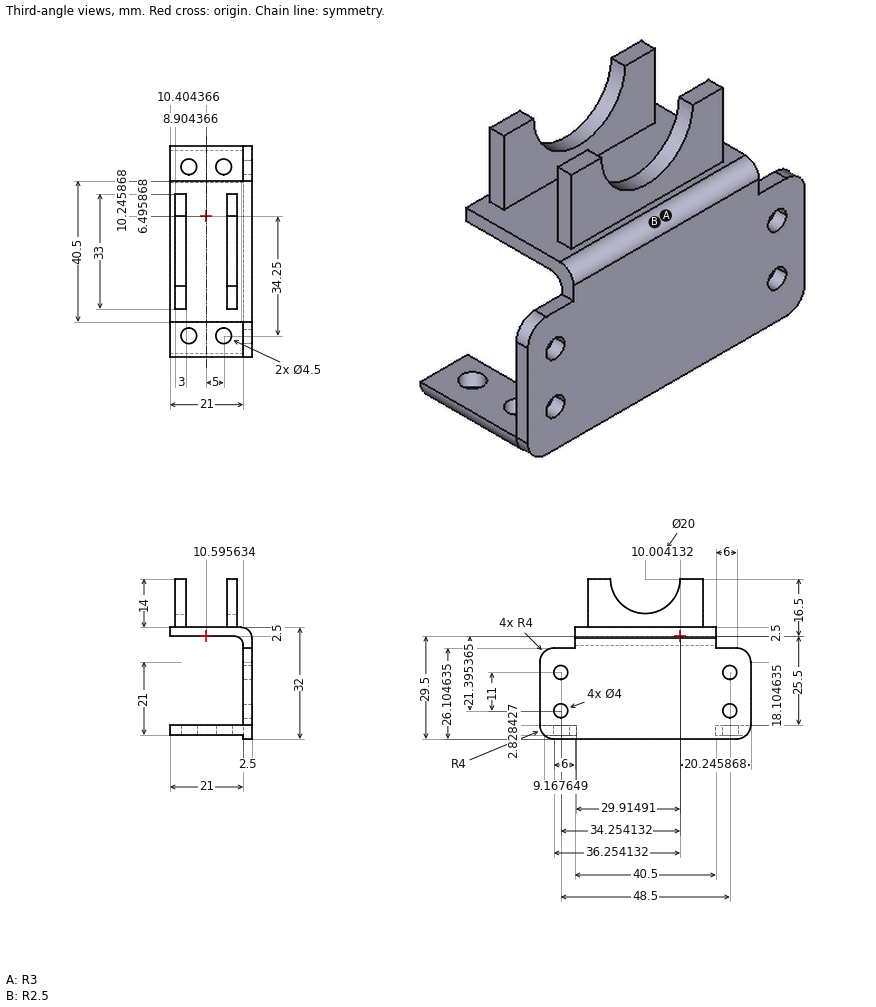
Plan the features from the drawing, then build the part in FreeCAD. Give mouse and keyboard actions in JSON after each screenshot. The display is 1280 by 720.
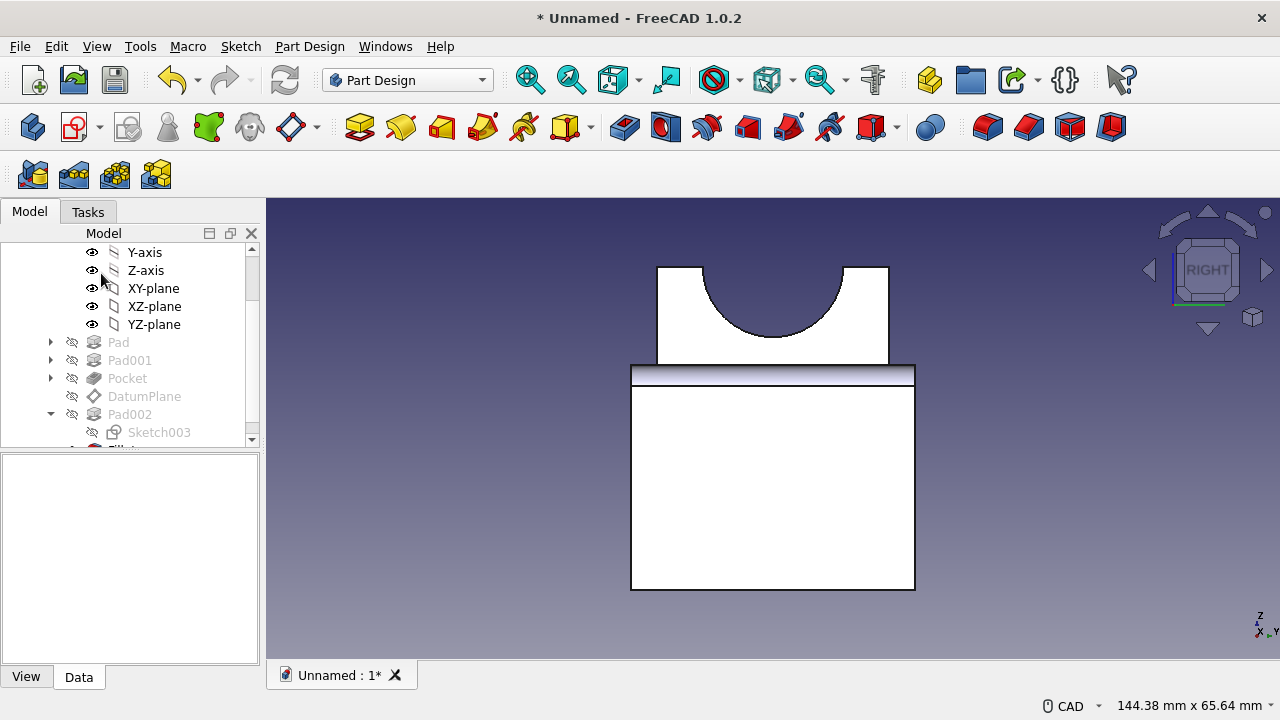
{"action": "key", "text": "5"}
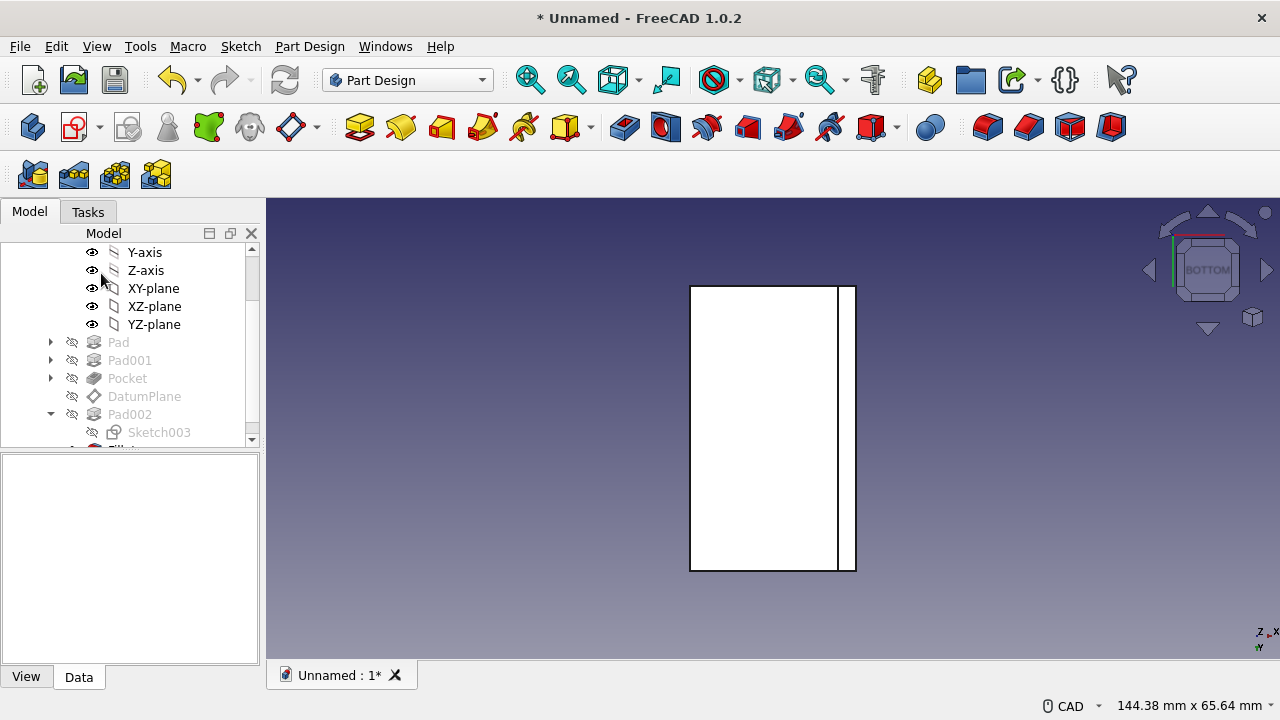
{"action": "key", "text": "4"}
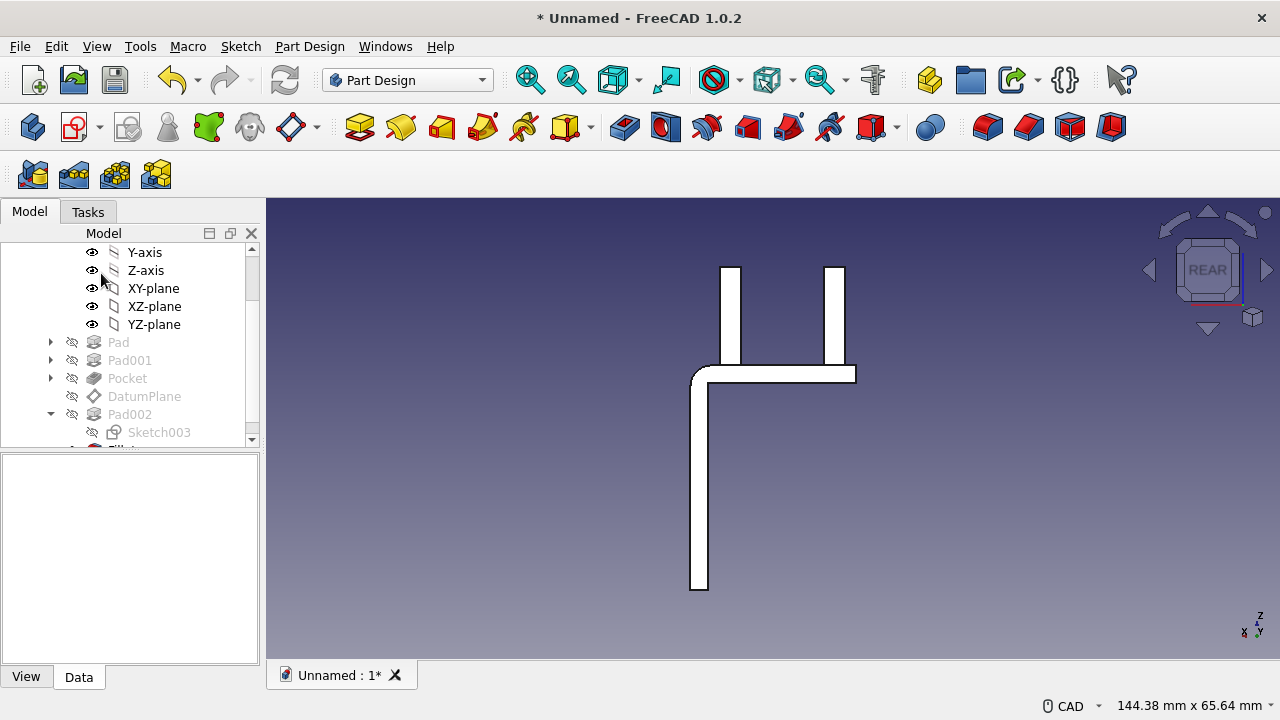
{"action": "key", "text": "6"}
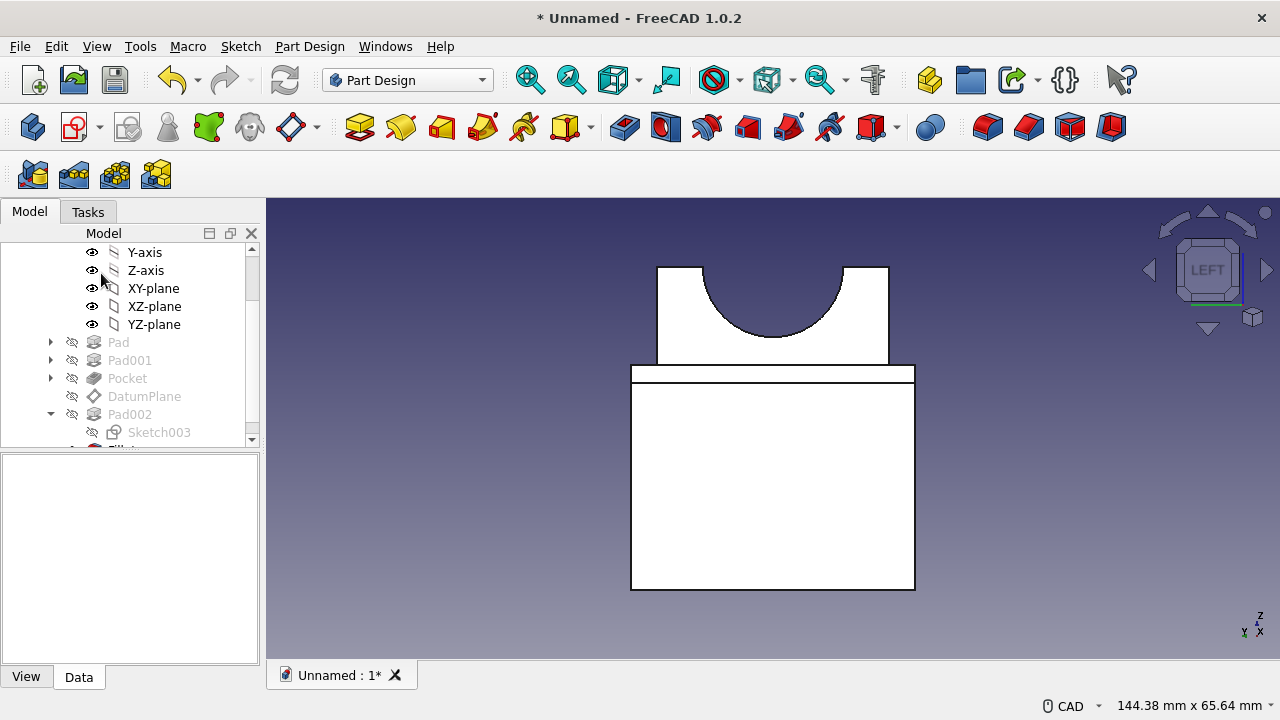
{"action": "key", "text": "v 3"}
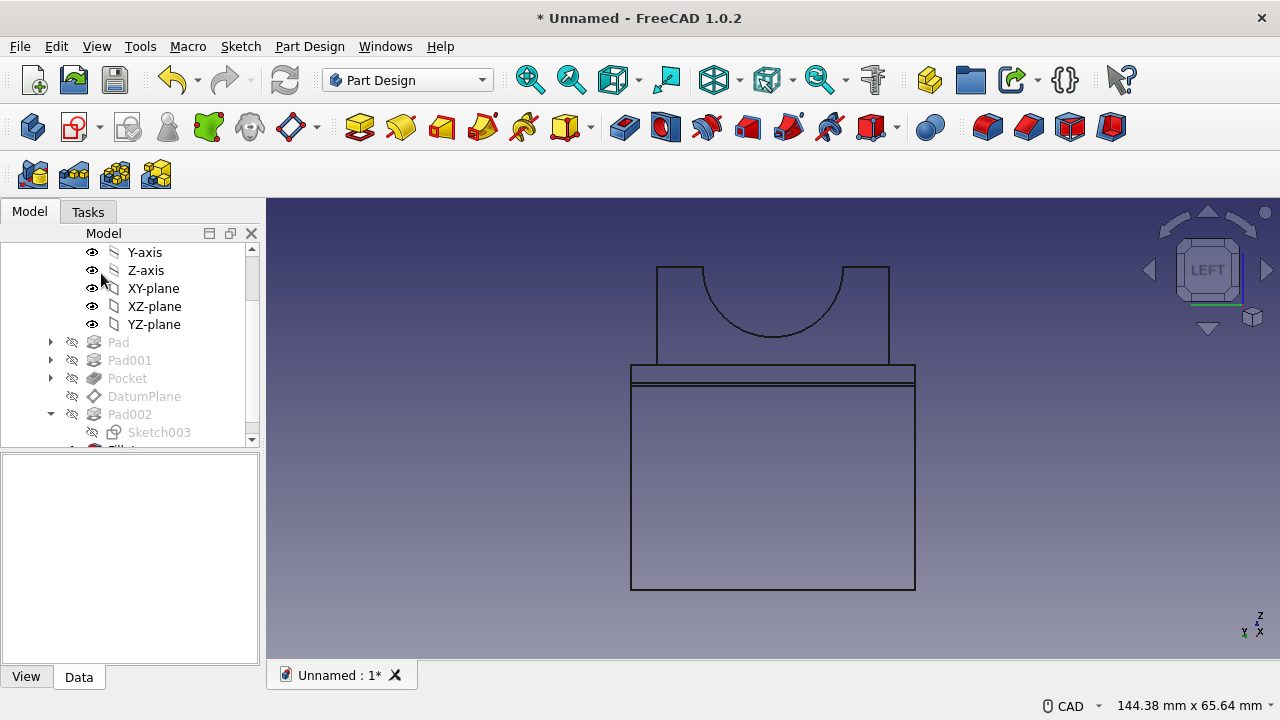
{"action": "key", "text": "0"}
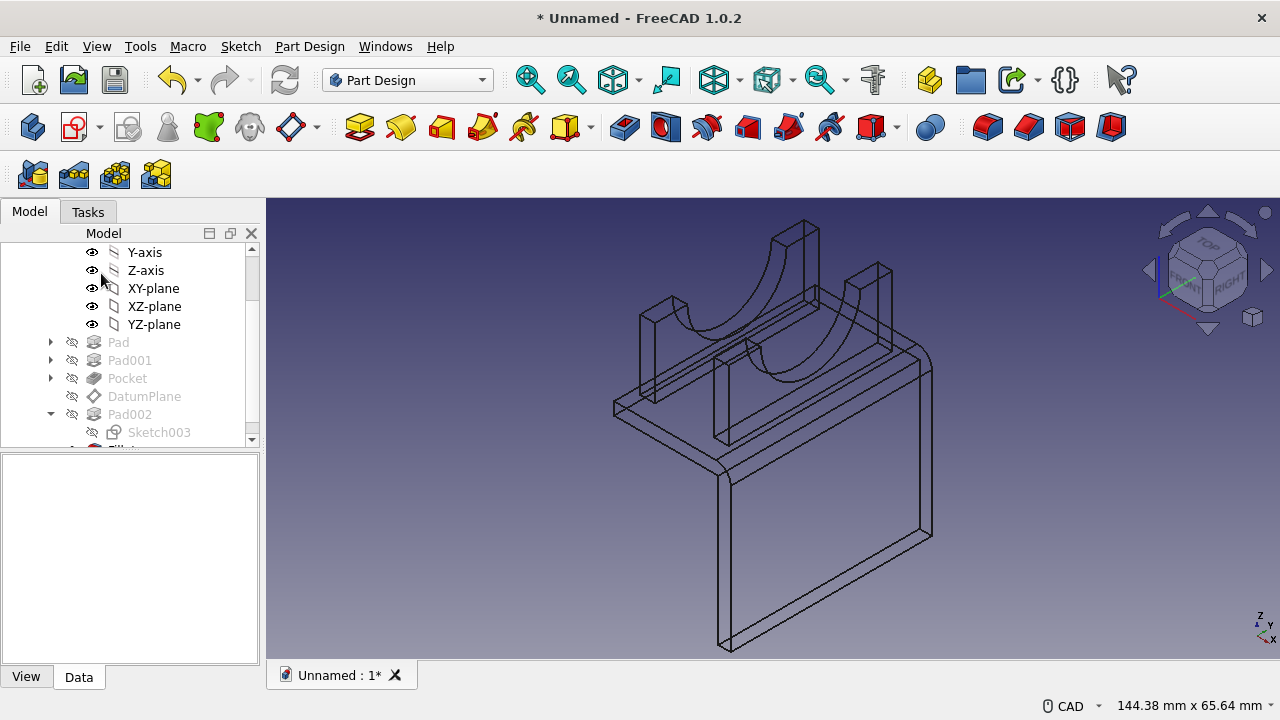
{"action": "left_click", "coordinate": [819, 417]}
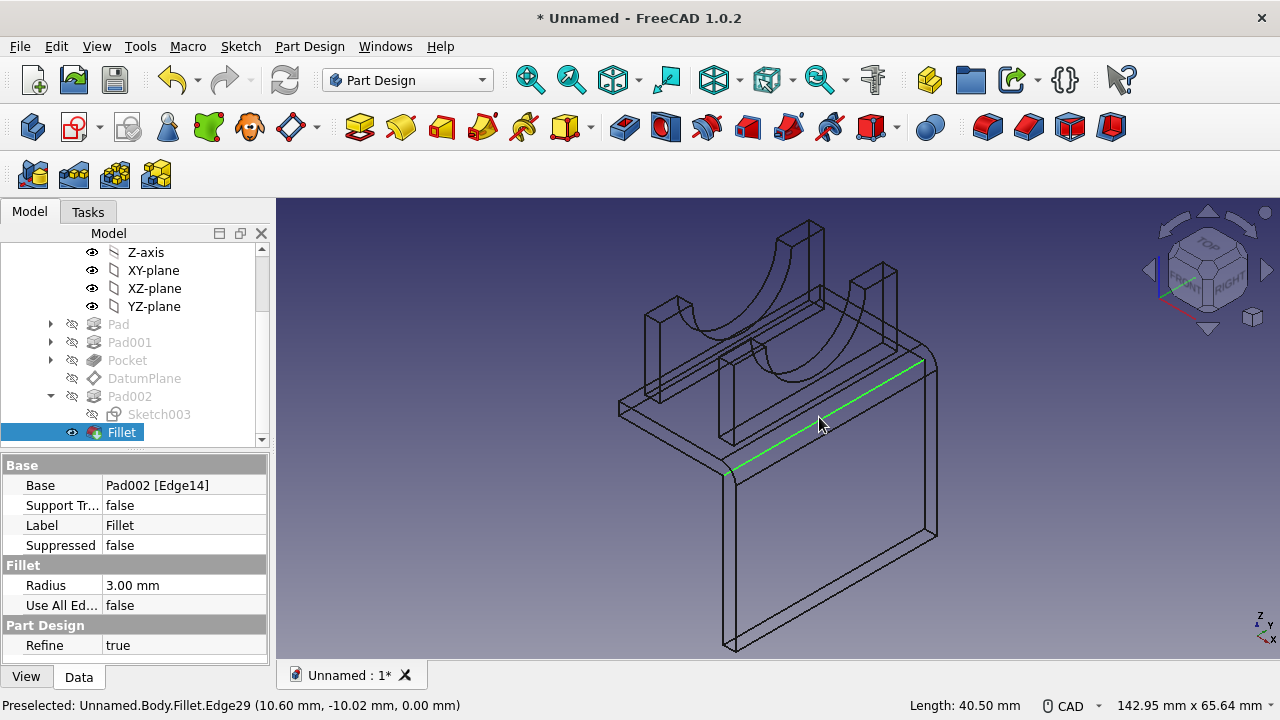
{"action": "key", "text": "v 1"}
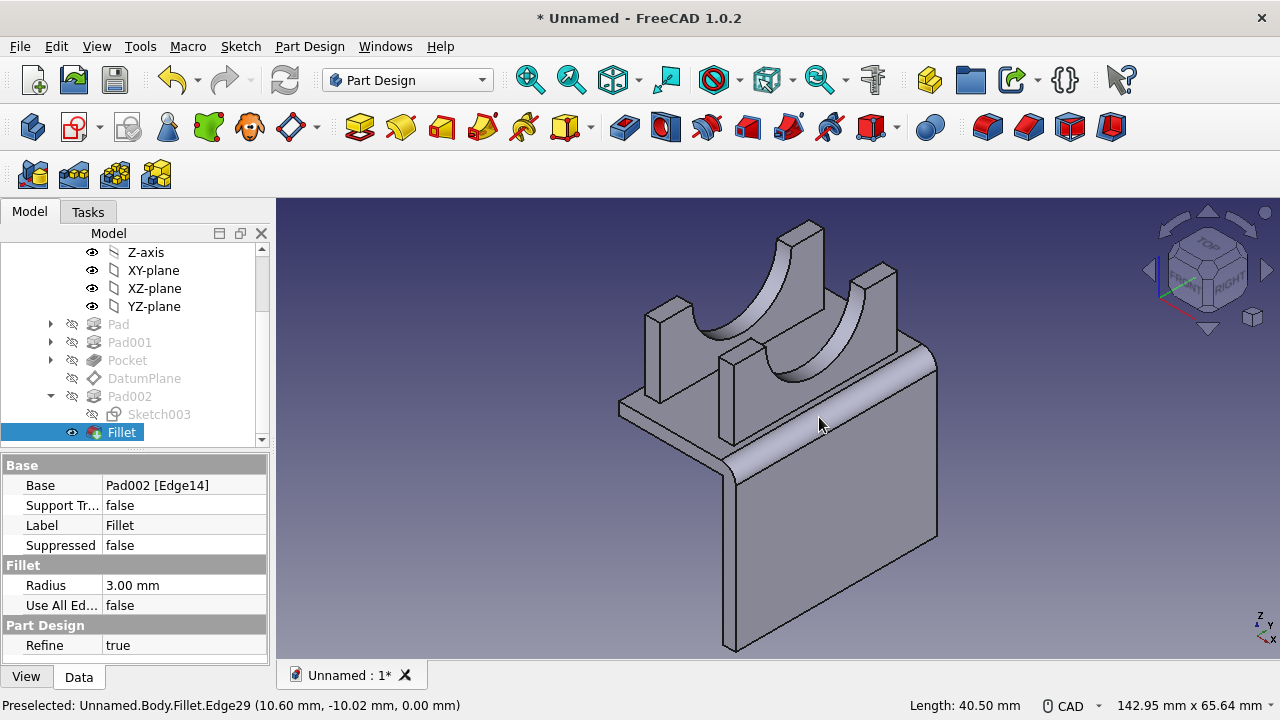
{"action": "left_click", "coordinate": [988, 128]}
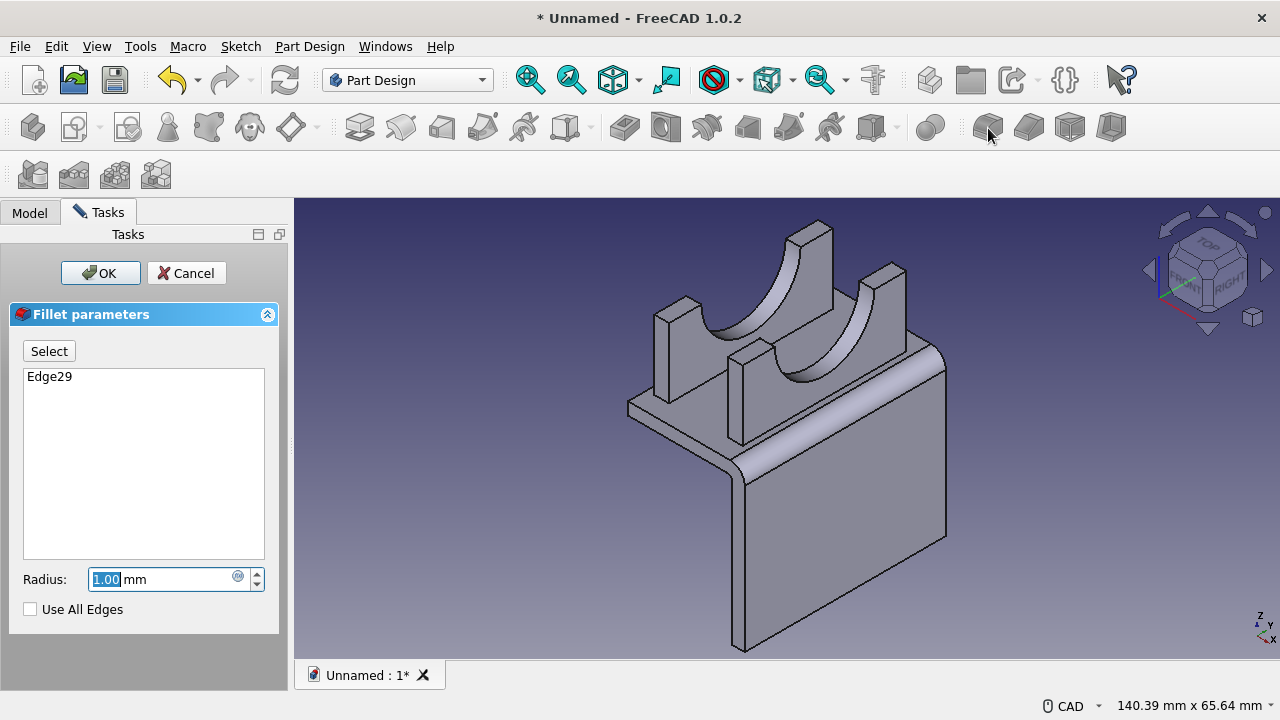
{"action": "type", "text": "2.5"}
{"action": "key", "text": "Tab"}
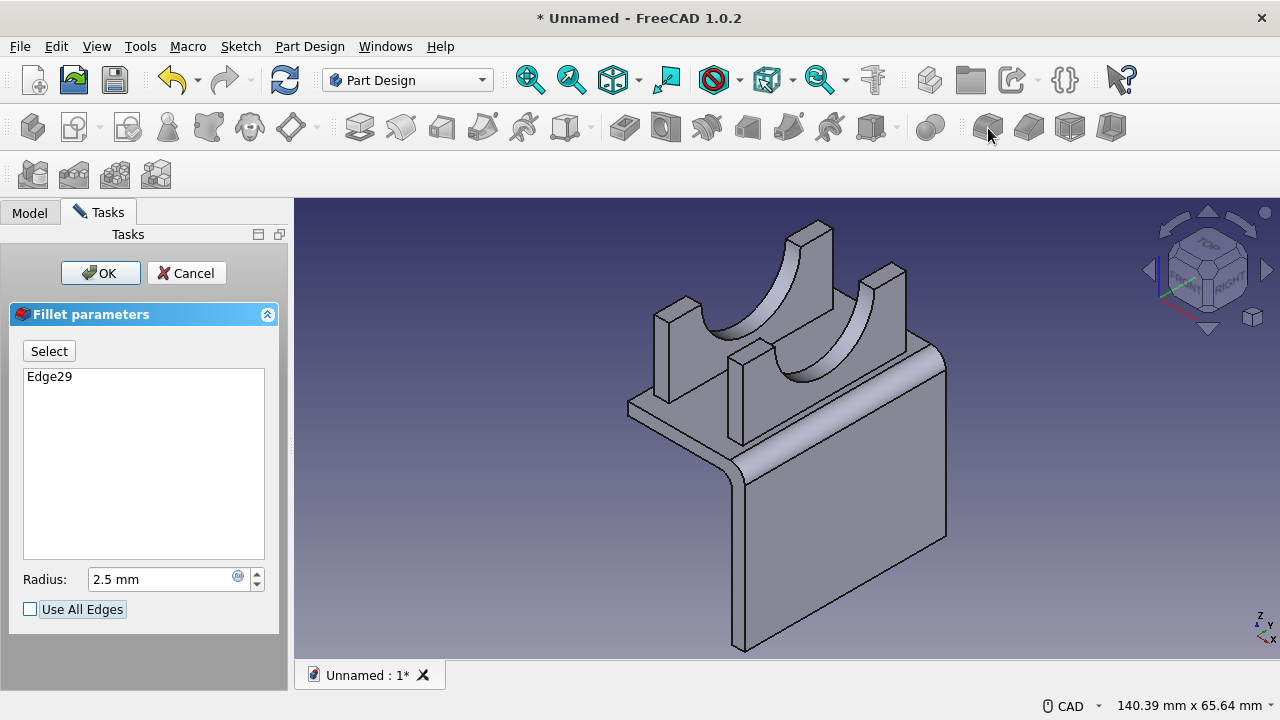
{"action": "left_click", "coordinate": [101, 273]}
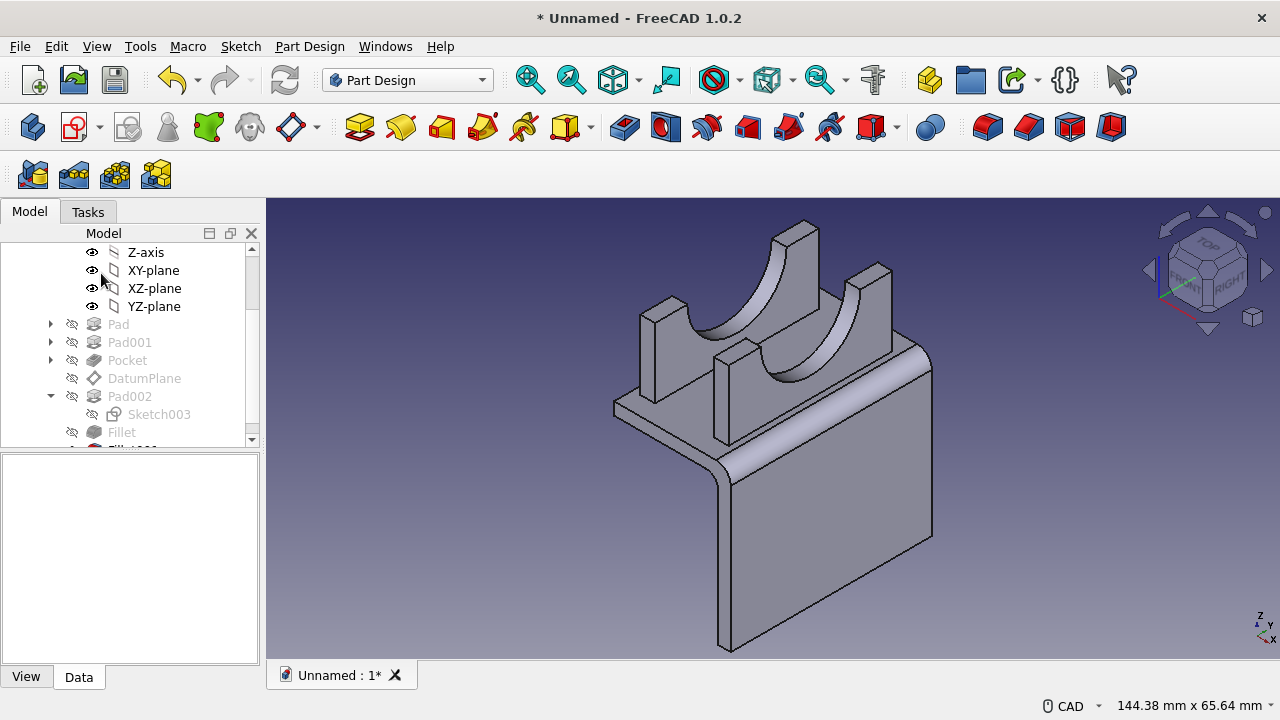
{"action": "left_click", "coordinate": [831, 510]}